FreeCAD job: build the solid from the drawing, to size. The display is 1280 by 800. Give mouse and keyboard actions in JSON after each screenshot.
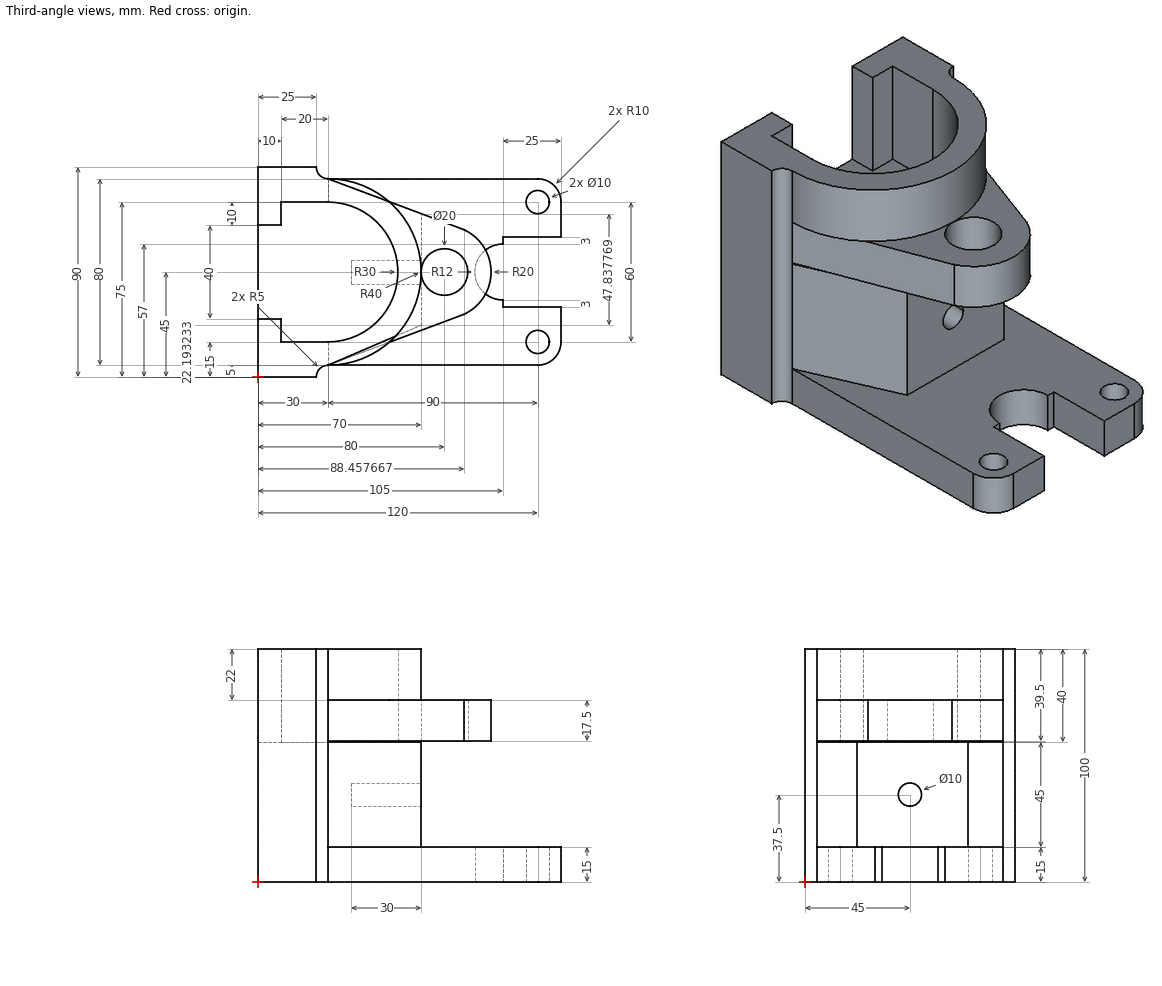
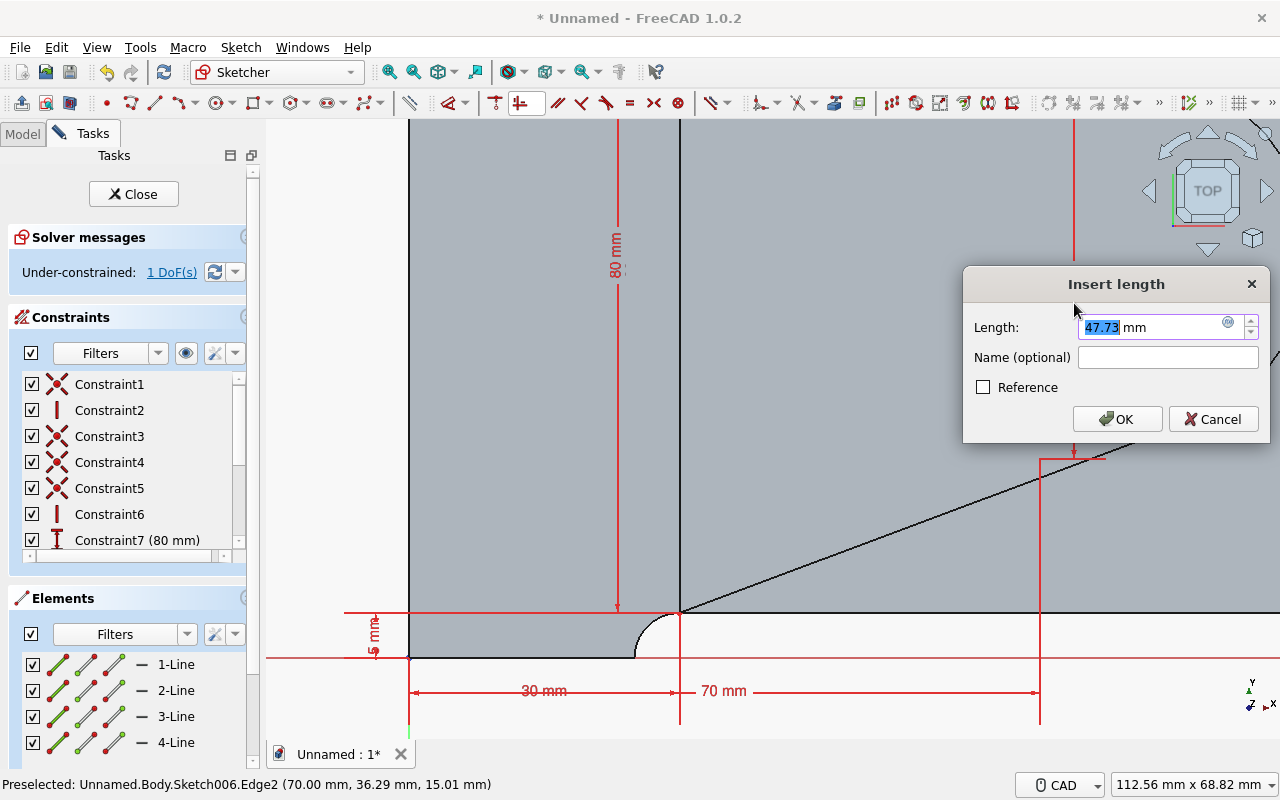
{"action": "type", "text": "47.837769"}
{"action": "key", "text": "Return"}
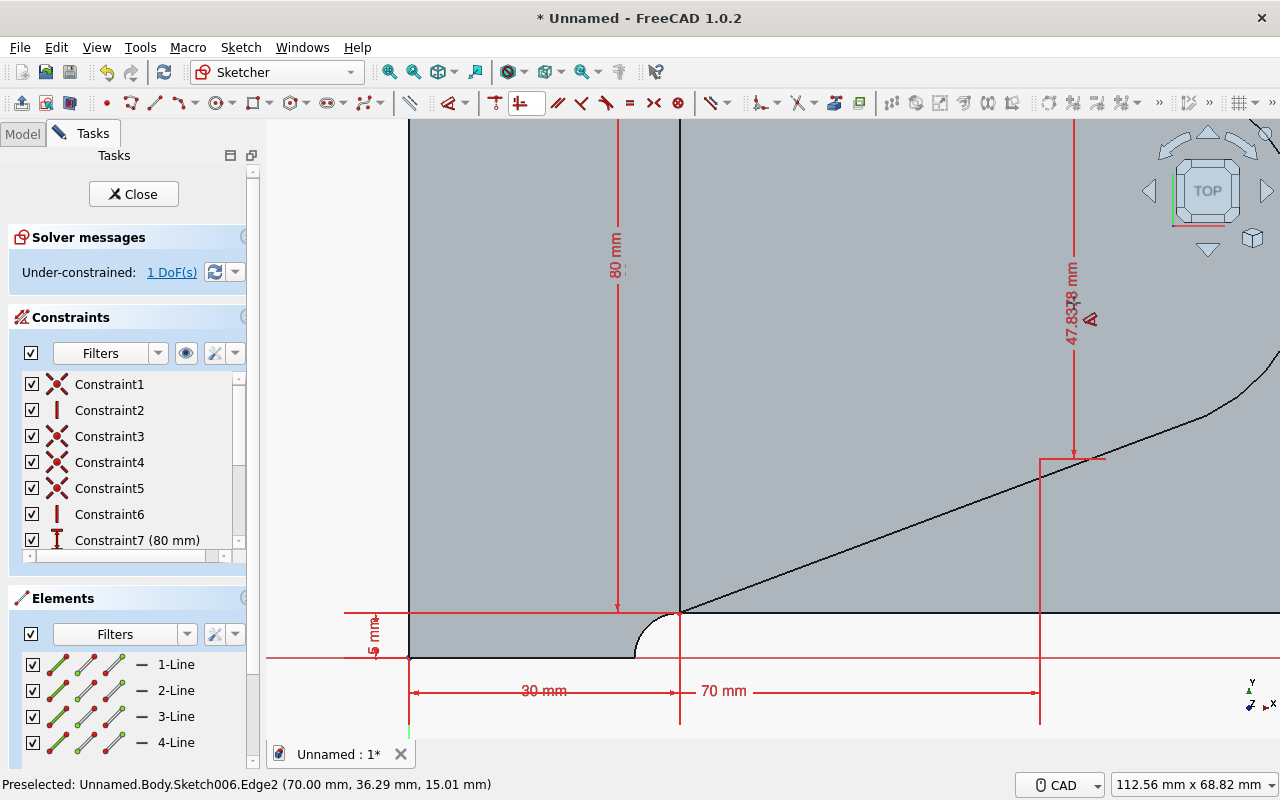
{"action": "left_click", "coordinate": [1040, 459]}
{"action": "left_click", "coordinate": [1074, 559]}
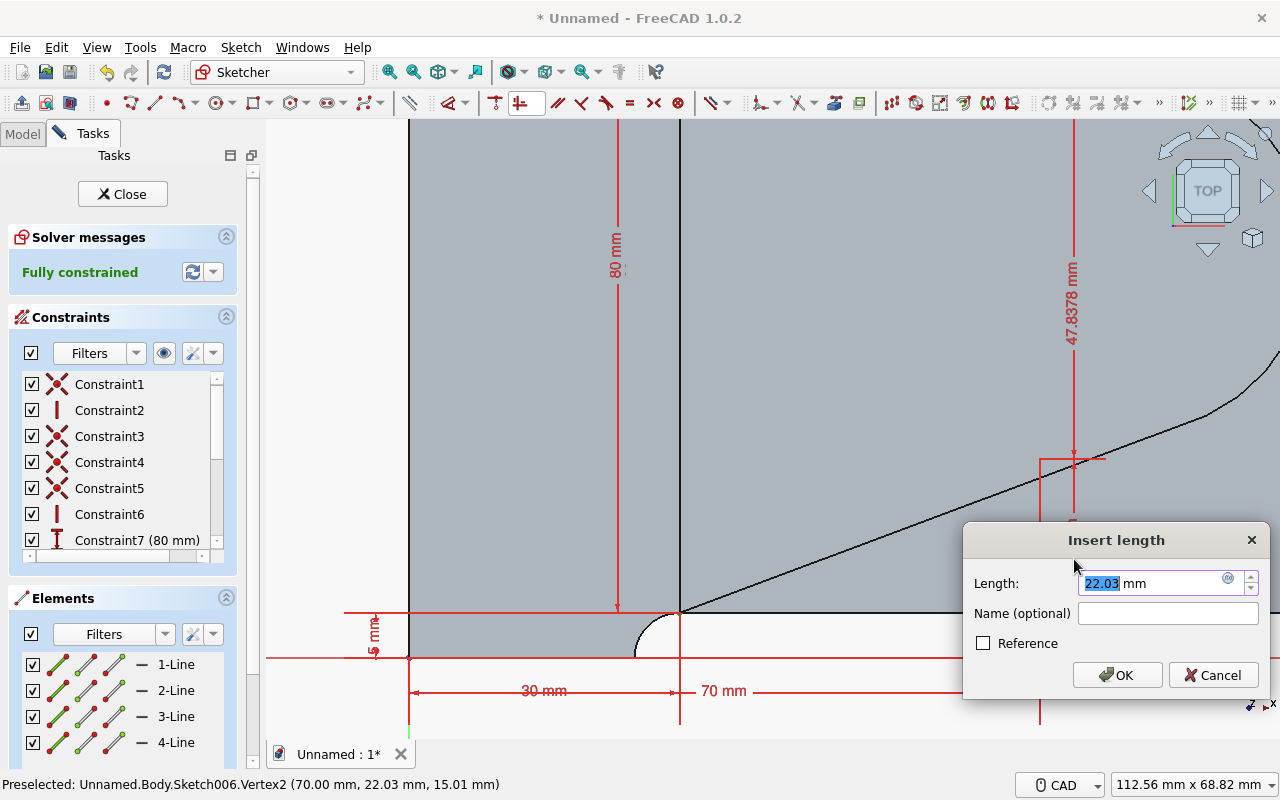
{"action": "type", "text": "22.193233"}
{"action": "key", "text": "Return"}
{"action": "key", "text": "Escape"}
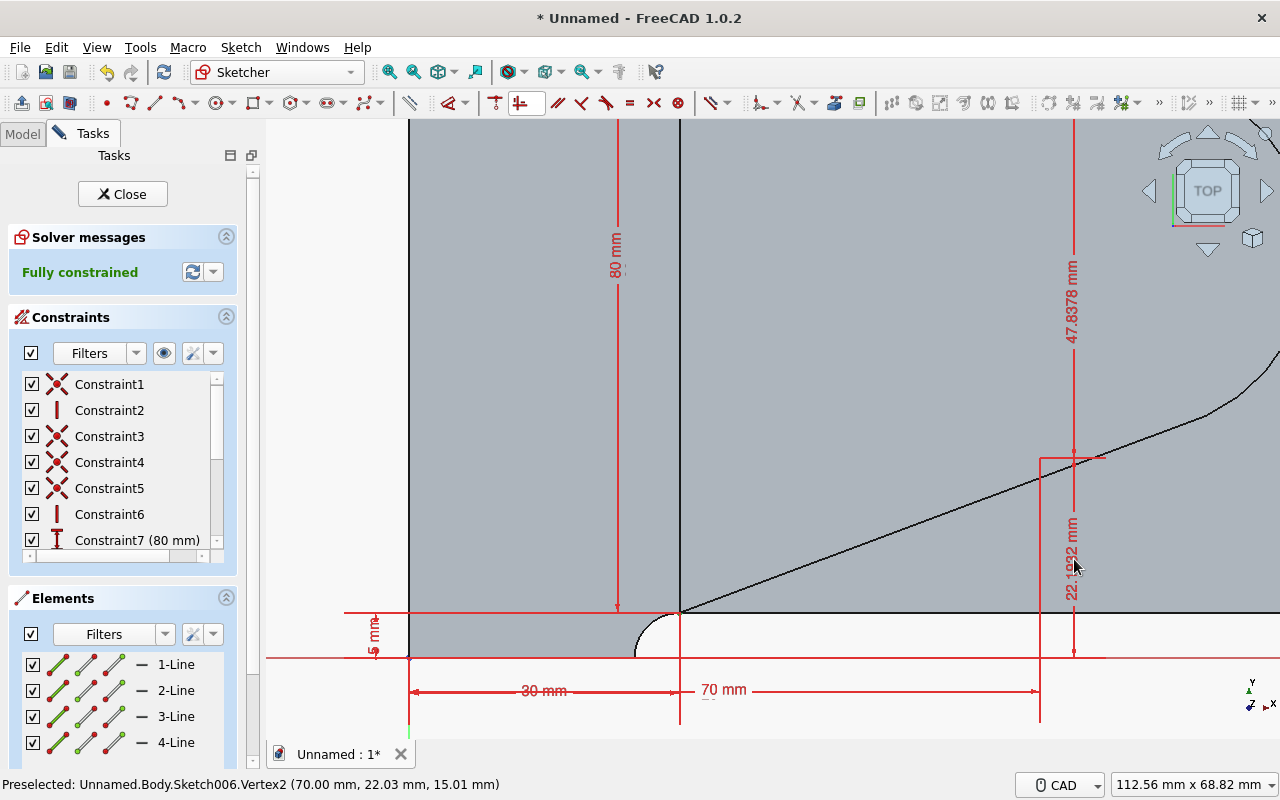
{"action": "left_click", "coordinate": [123, 194]}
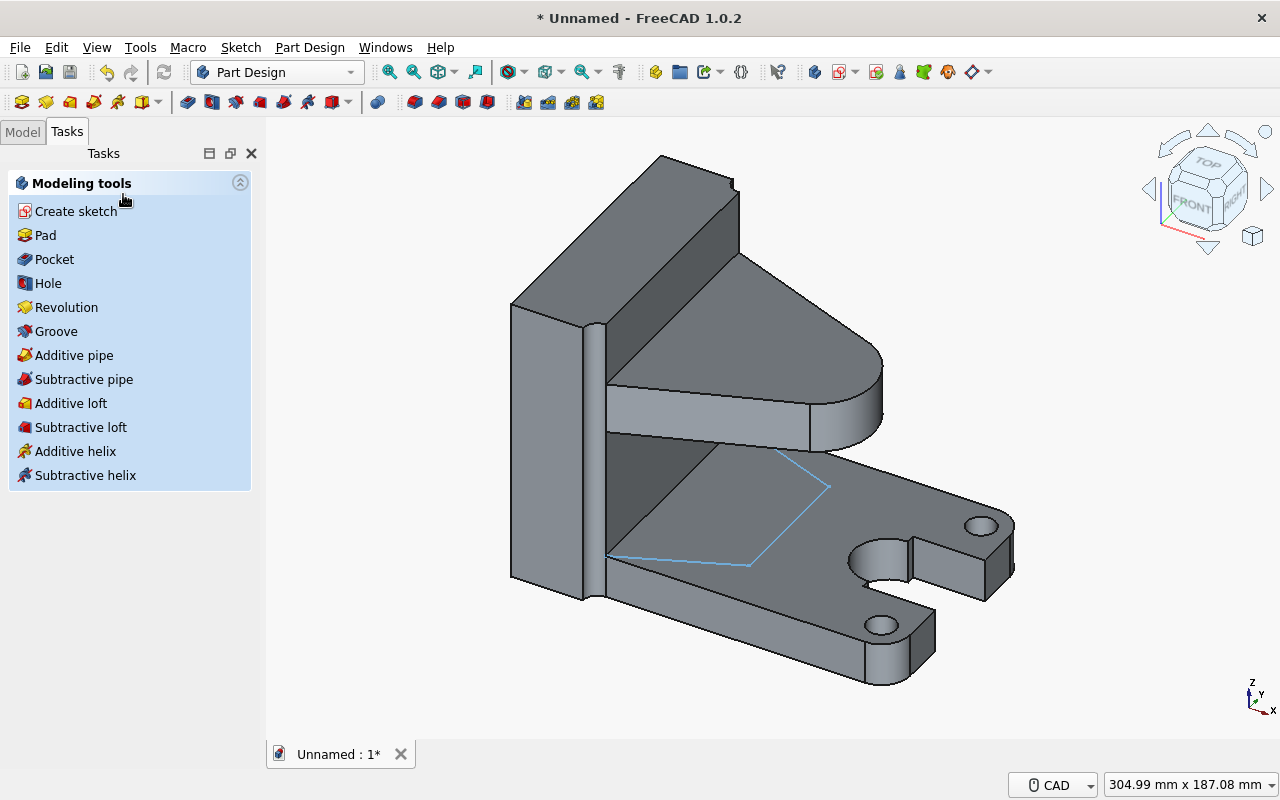
{"action": "left_click", "coordinate": [22, 102]}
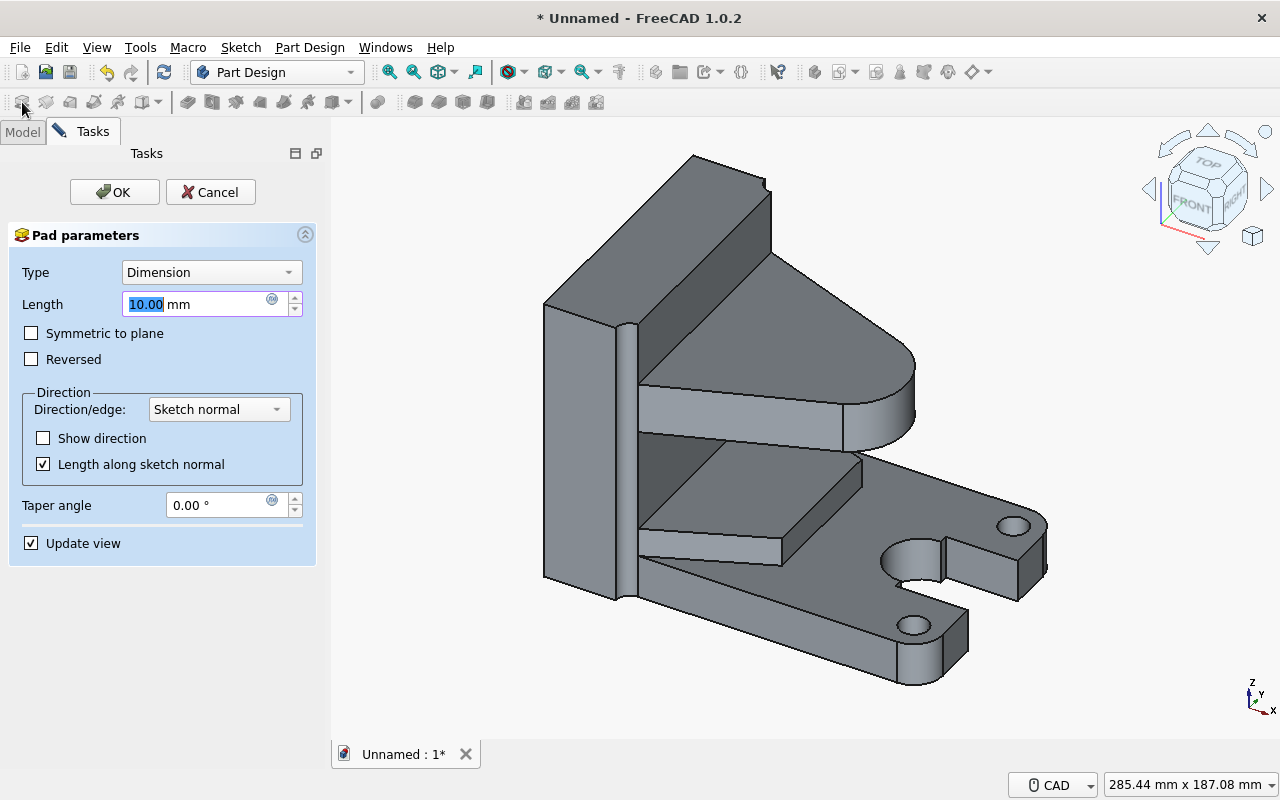
{"action": "type", "text": "45"}
{"action": "key", "text": "Tab"}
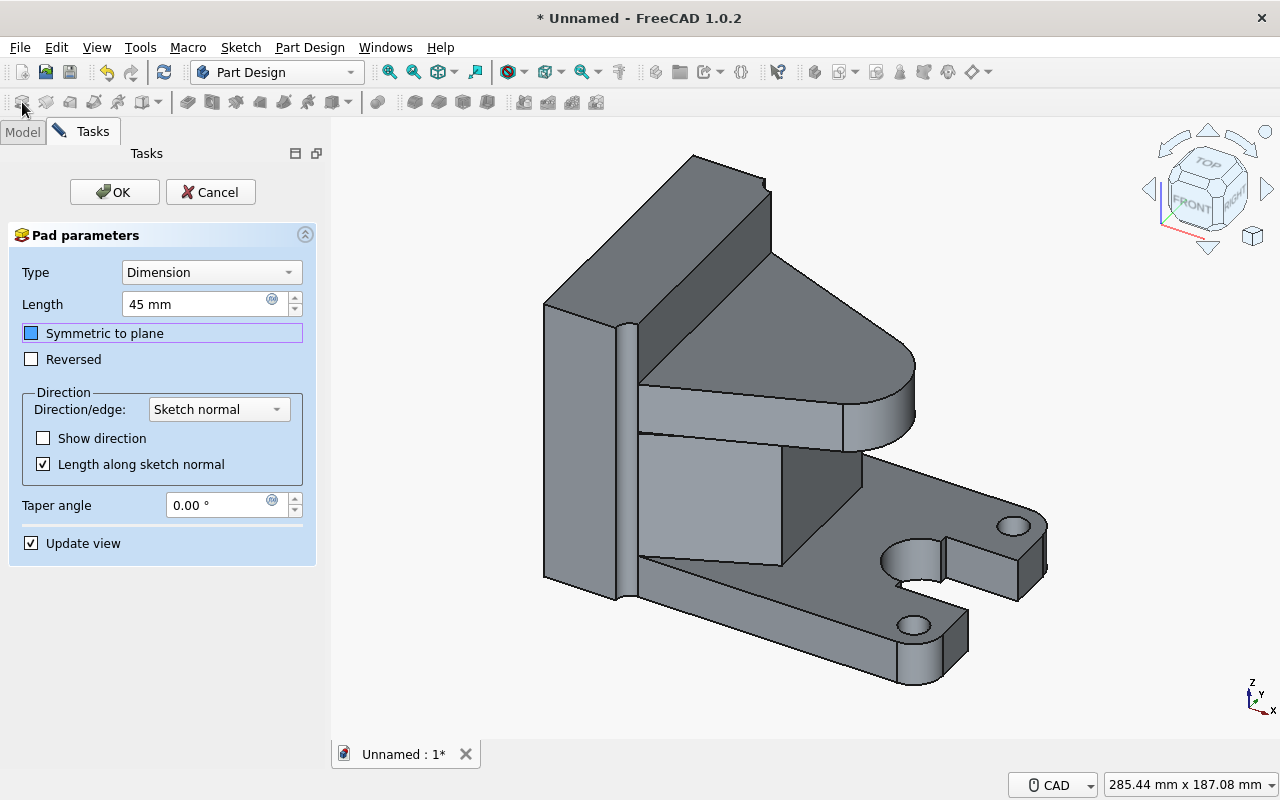
{"action": "left_click", "coordinate": [115, 192]}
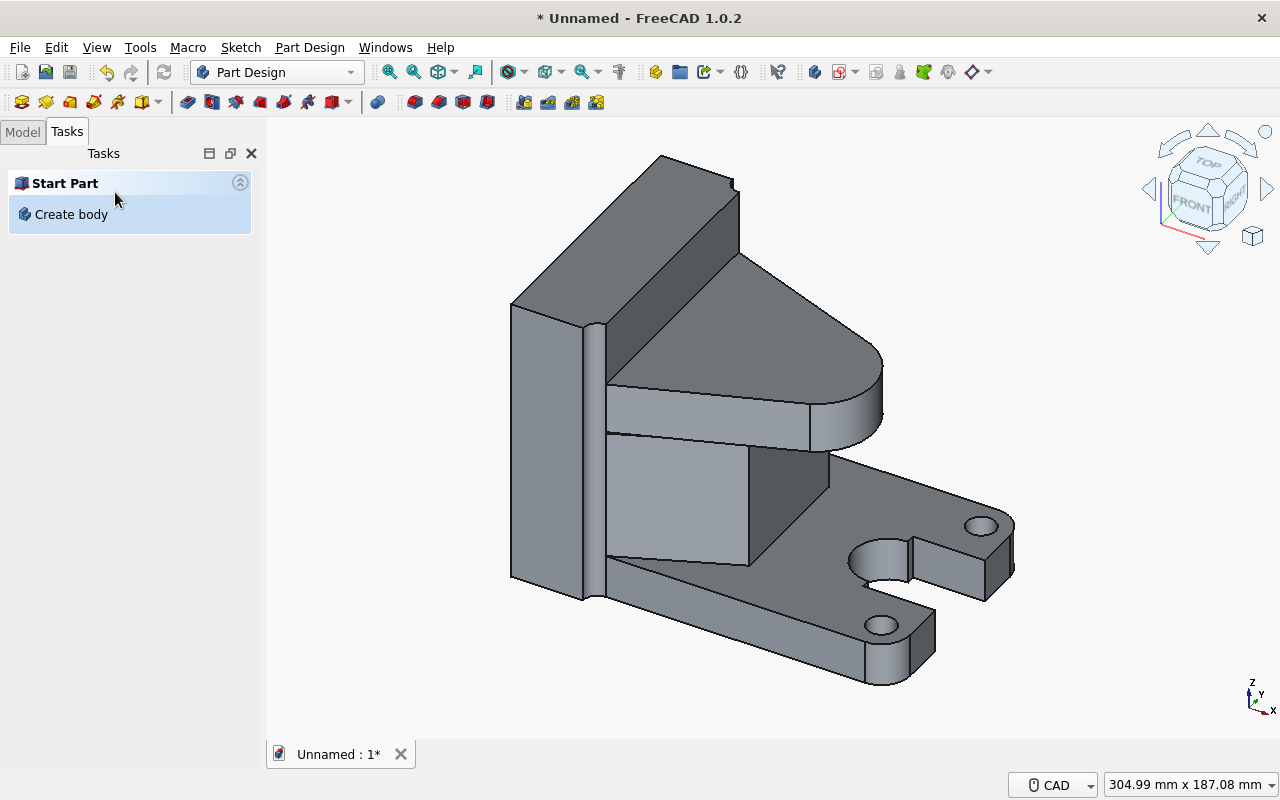
{"action": "left_click", "coordinate": [773, 351]}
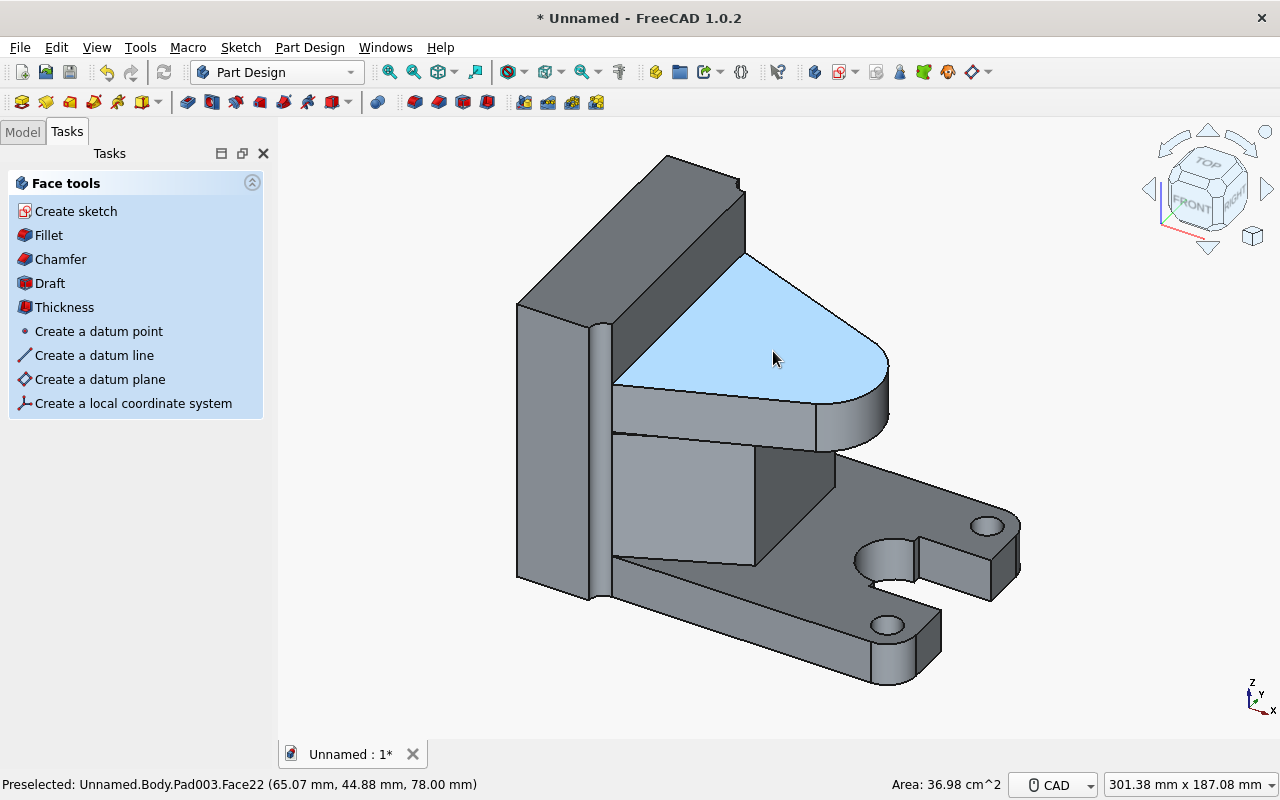
{"action": "left_click", "coordinate": [840, 72]}